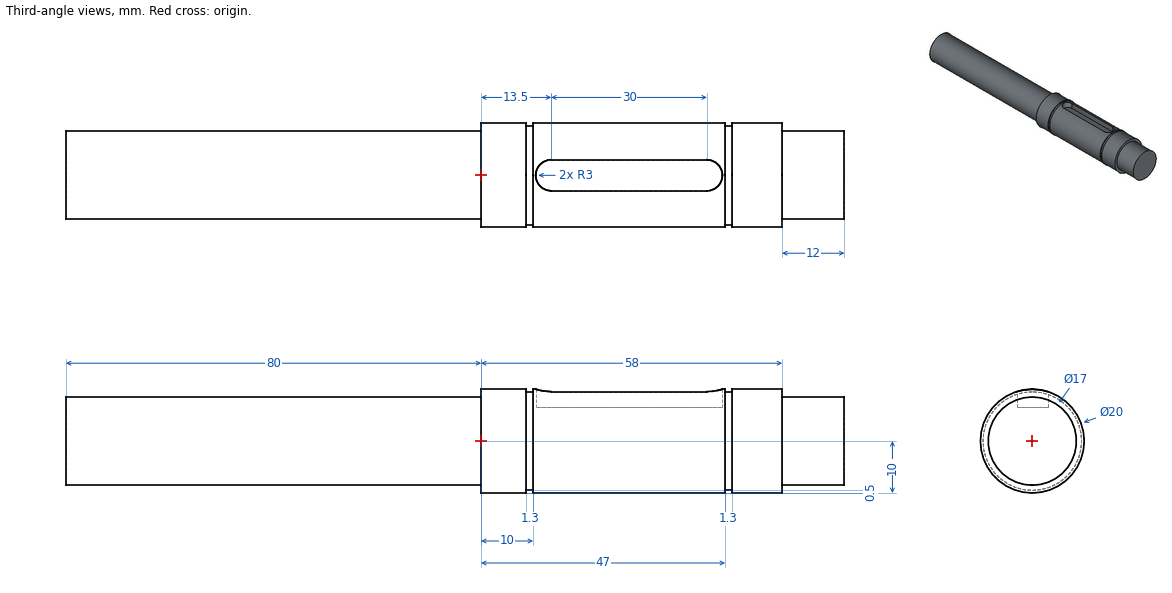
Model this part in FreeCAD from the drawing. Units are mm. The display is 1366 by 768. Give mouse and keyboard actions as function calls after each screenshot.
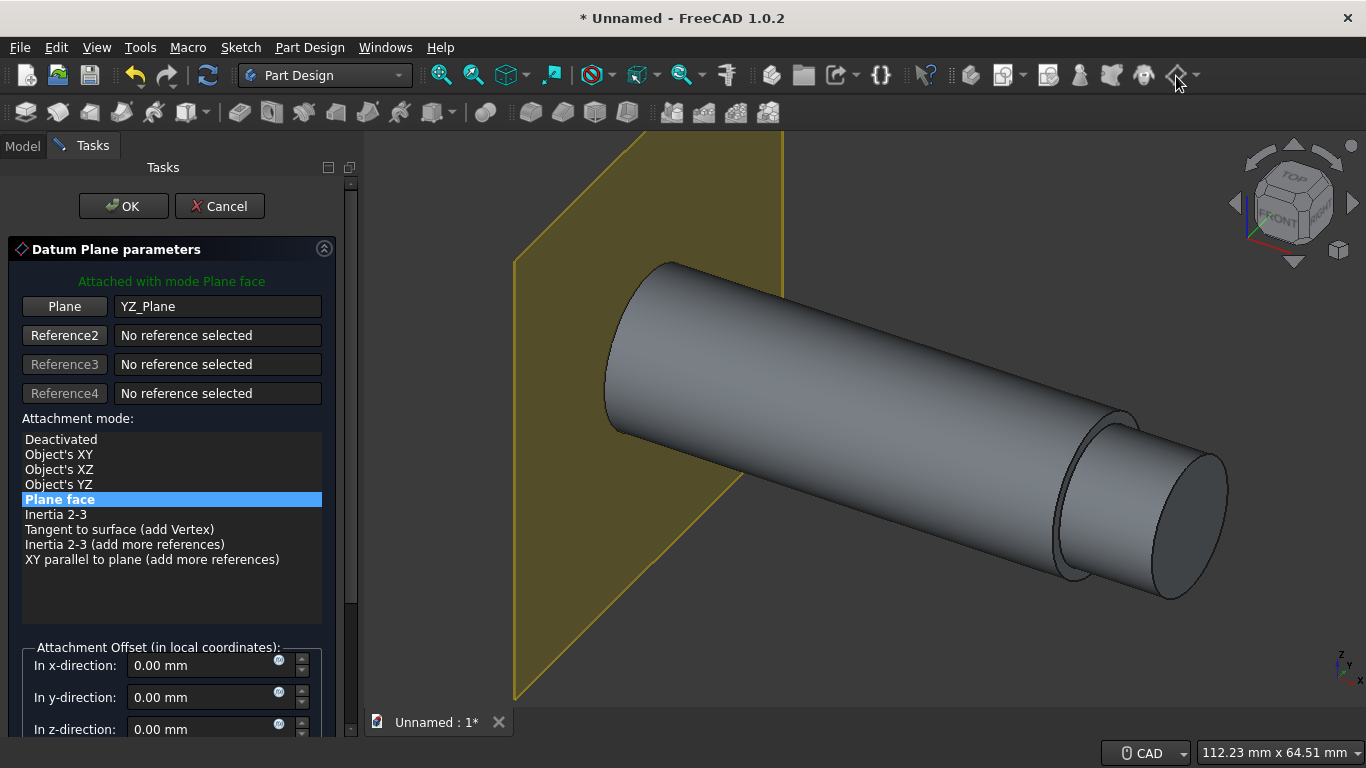
scroll(351, 456, down, 2)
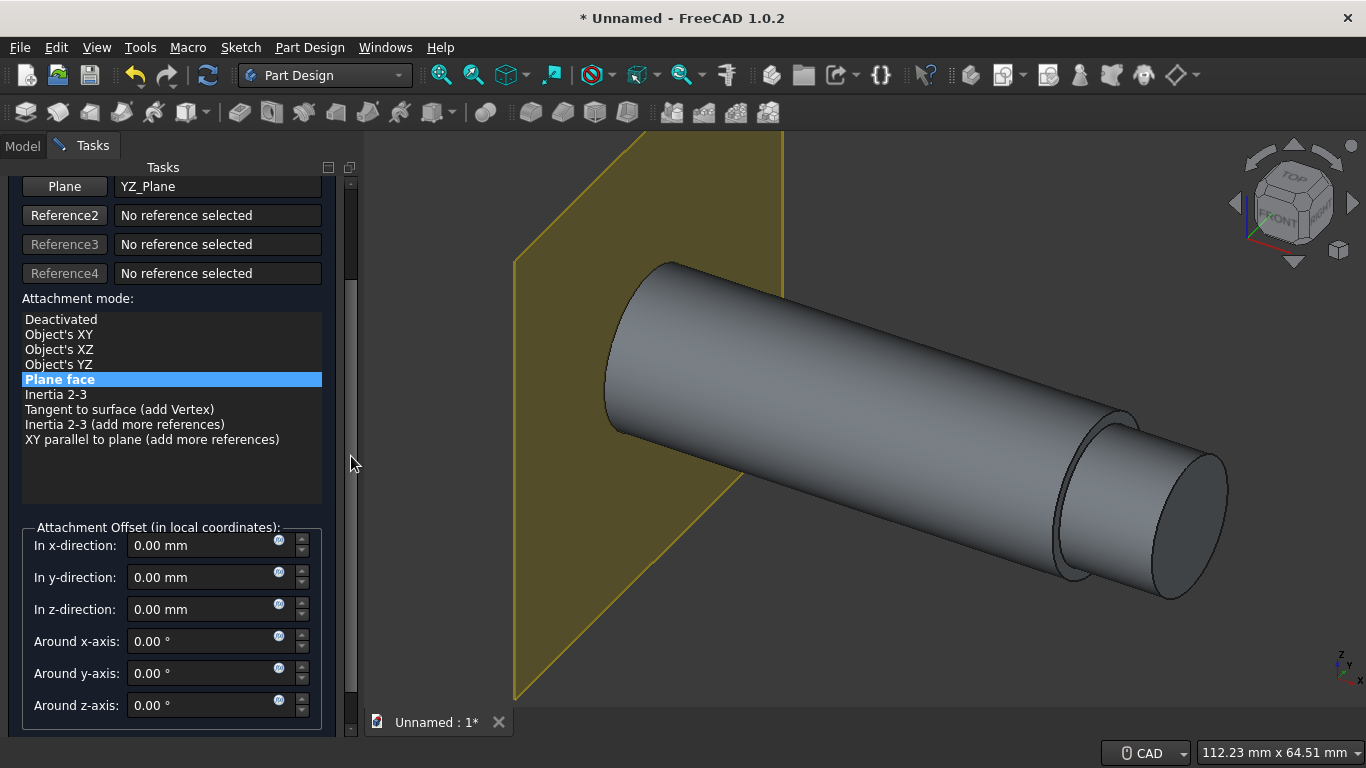
triple_click(210, 609)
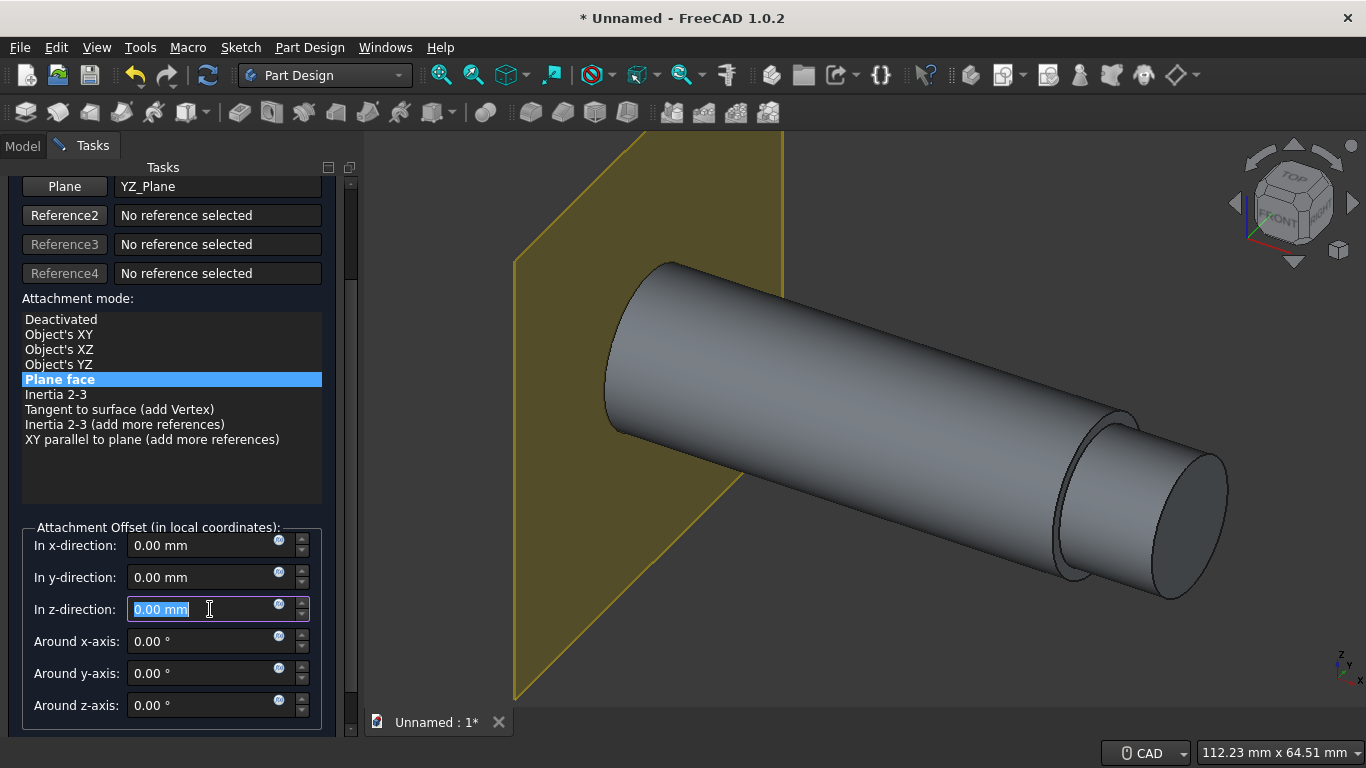
text(-80)
key(Tab)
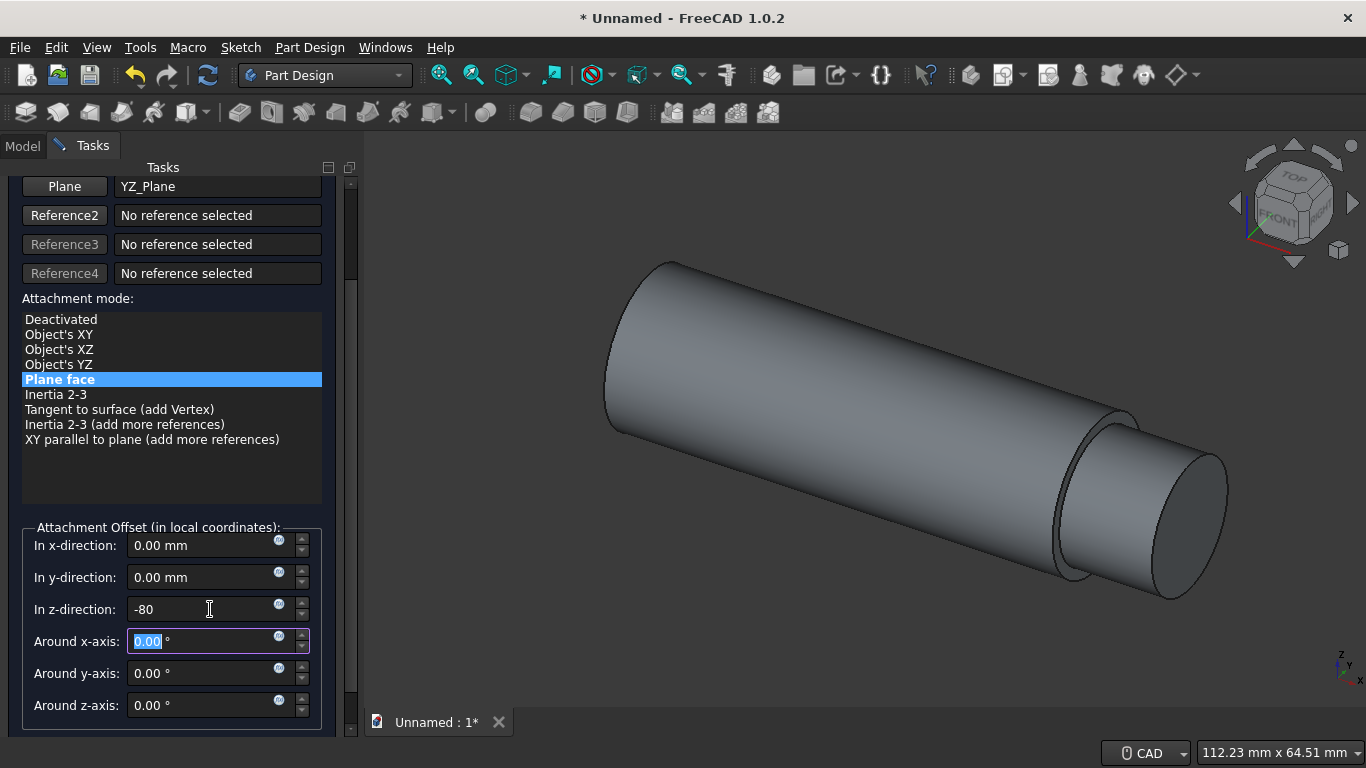
scroll(351, 456, up, 3)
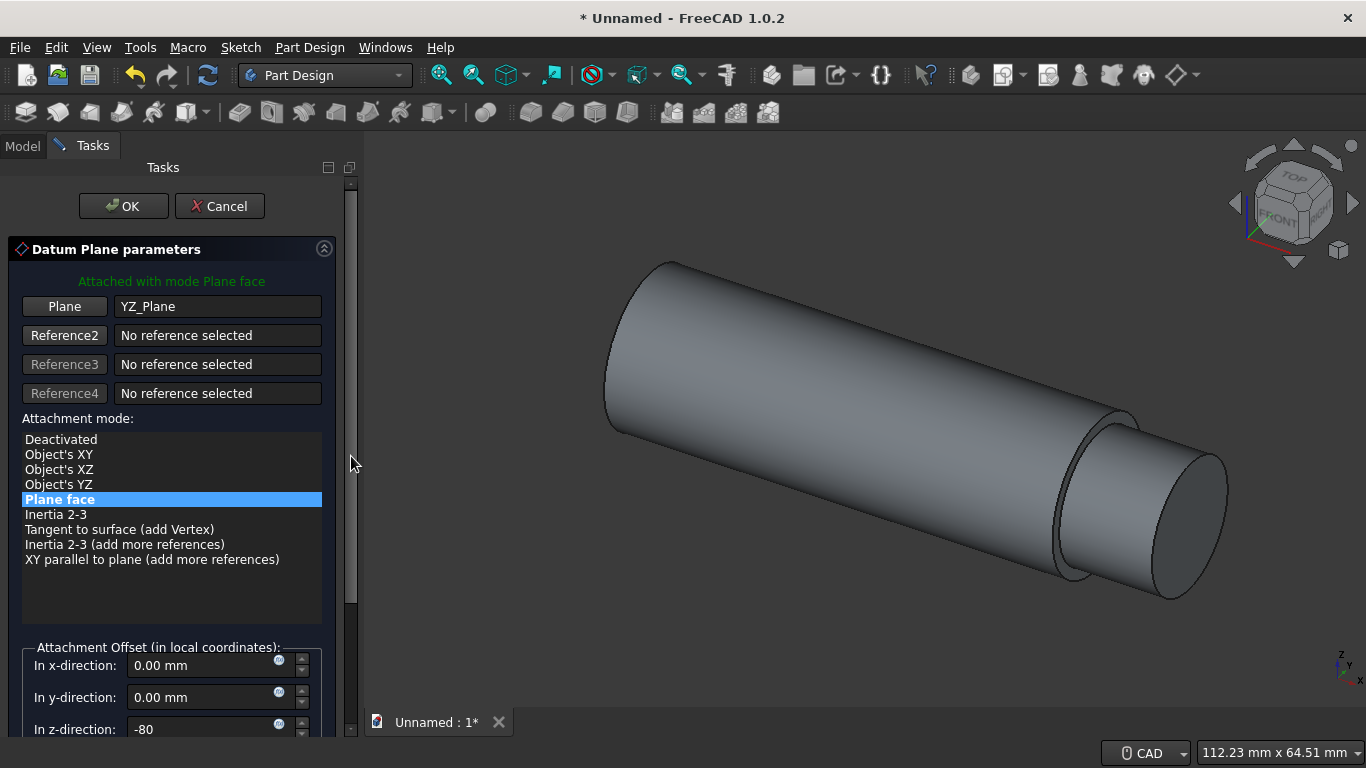
click(124, 206)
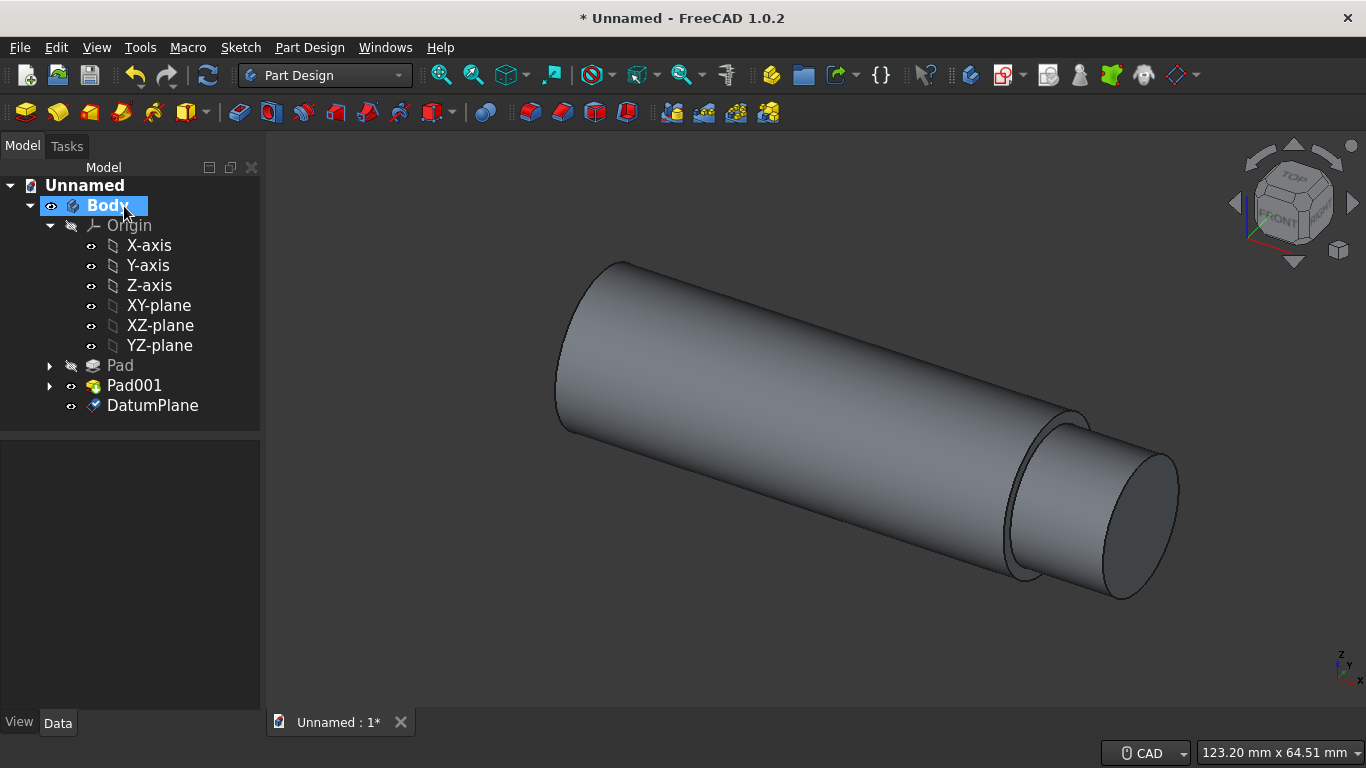
click(116, 406)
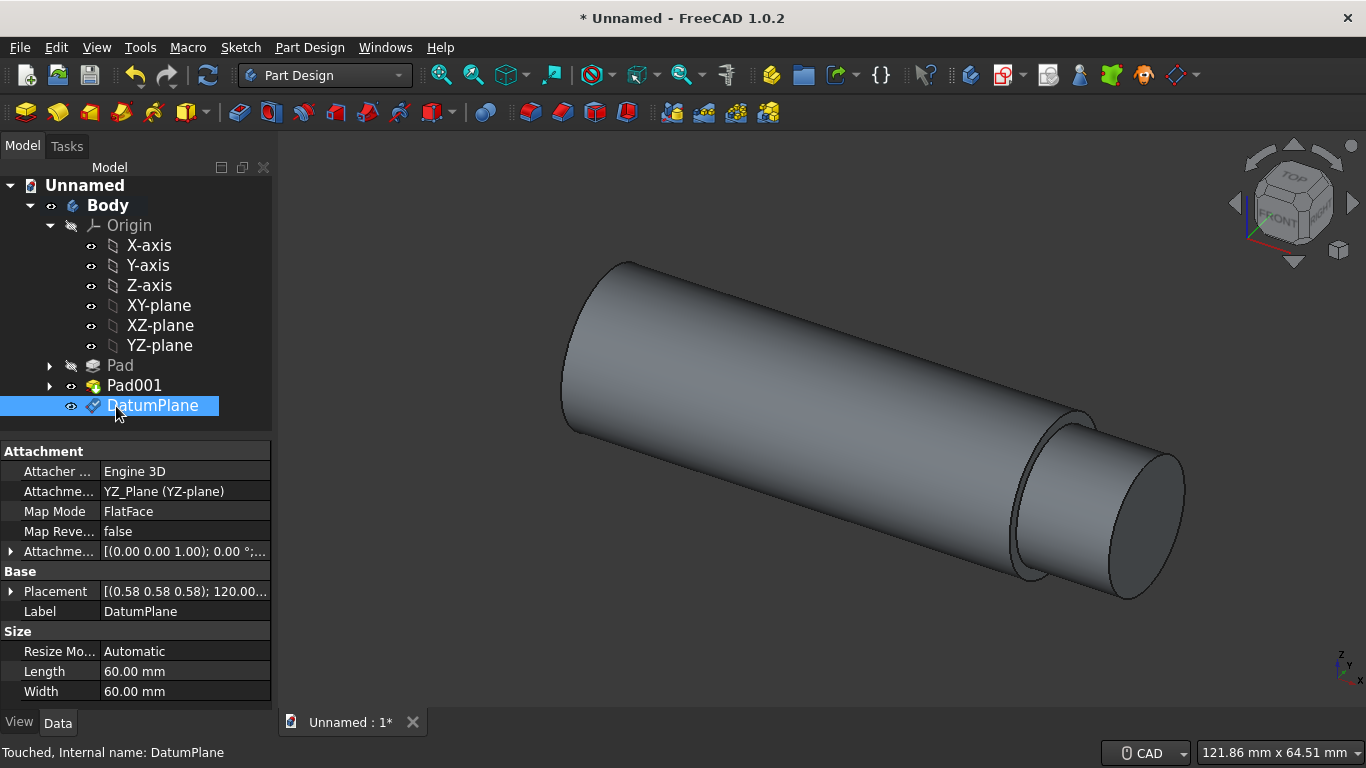
click(1004, 76)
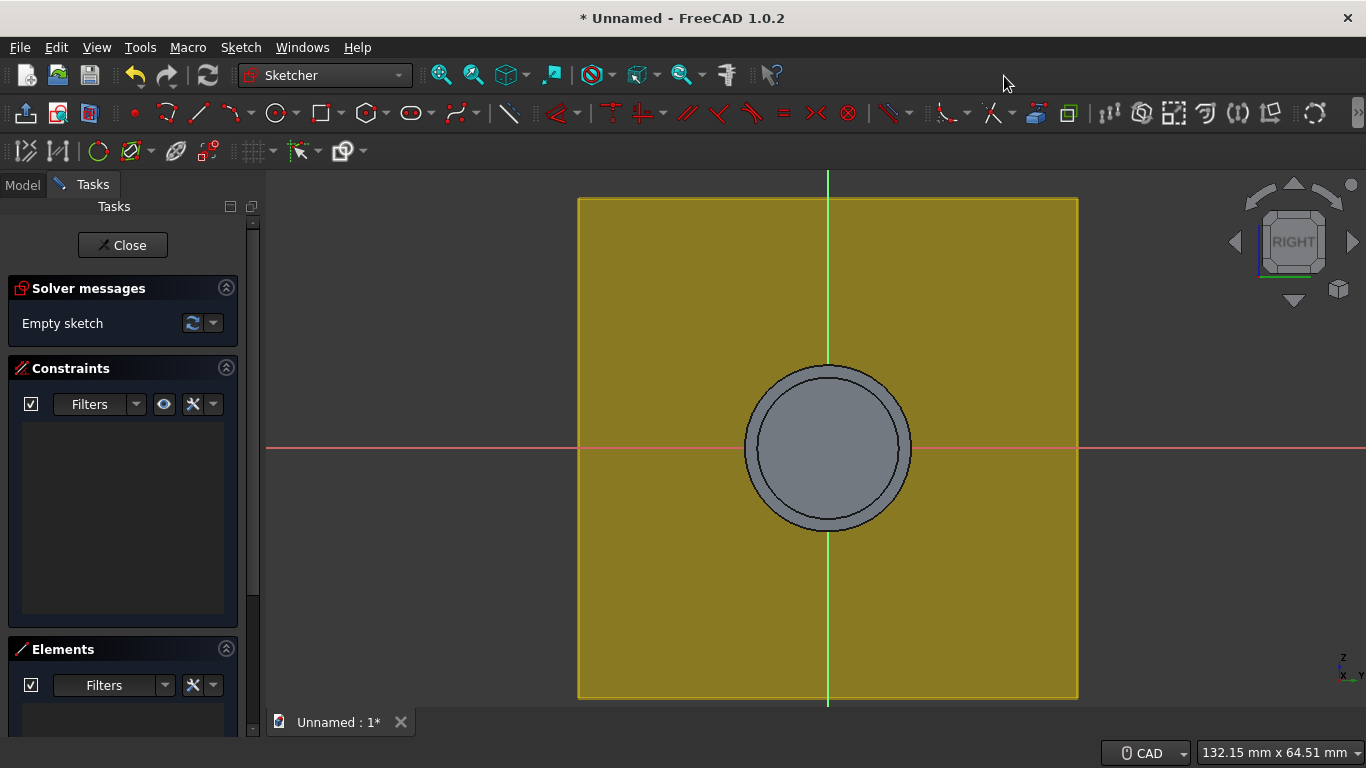
key(q)
key(s)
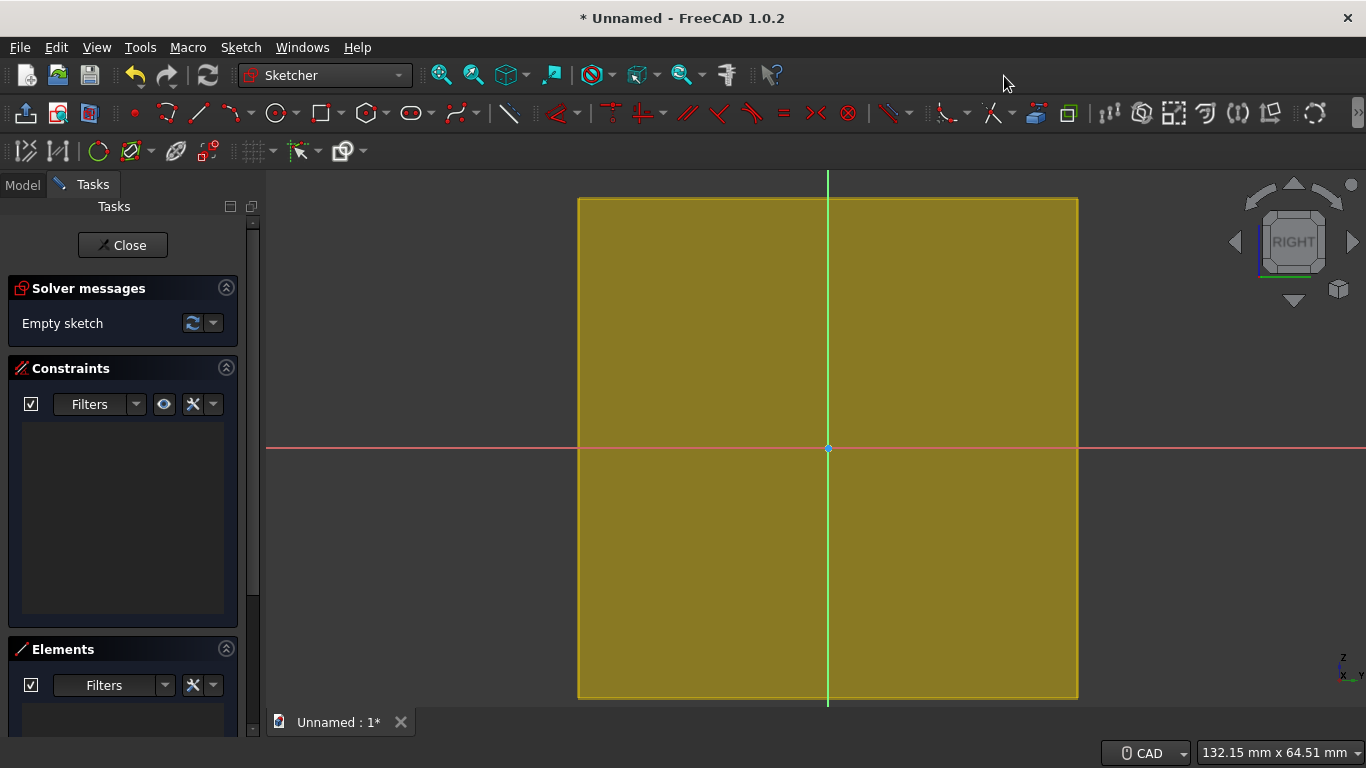
scroll(894, 456, up, 4)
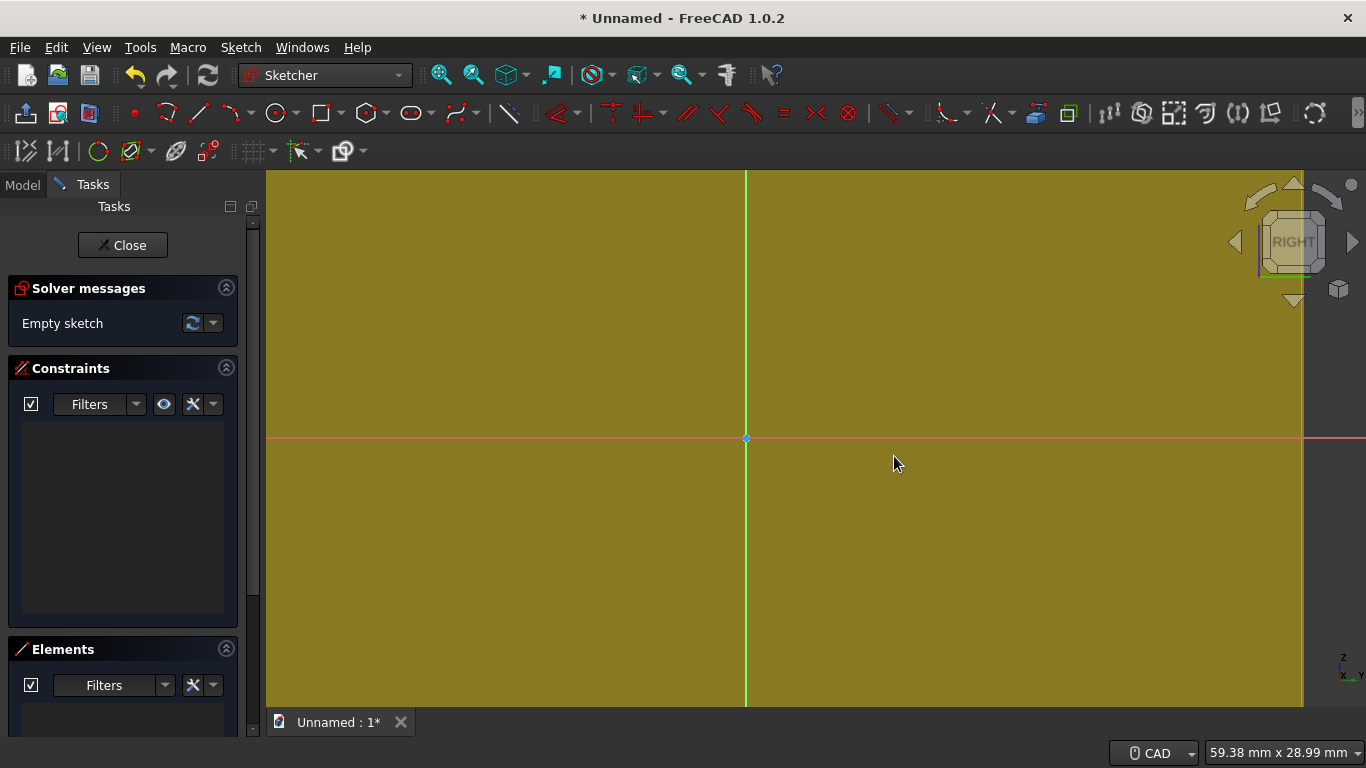
key(g)
key(c)